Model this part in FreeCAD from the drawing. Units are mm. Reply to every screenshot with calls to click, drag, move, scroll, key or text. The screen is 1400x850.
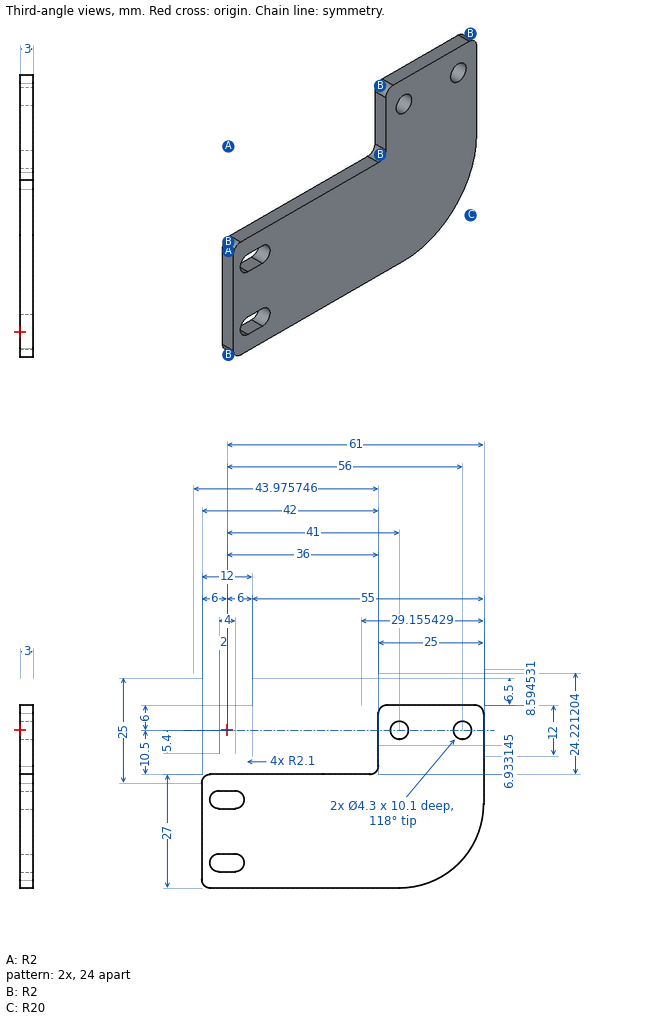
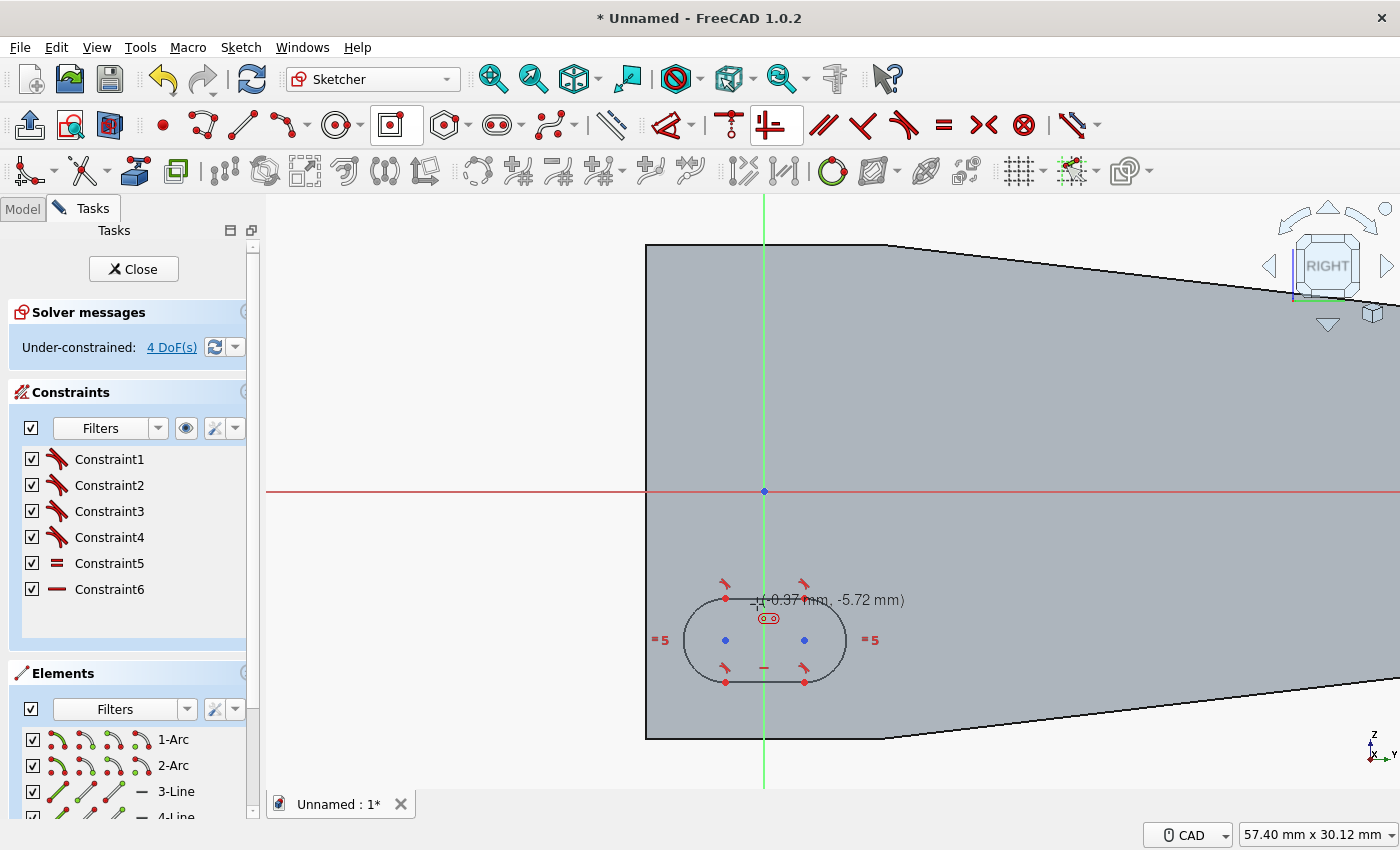
click(725, 344)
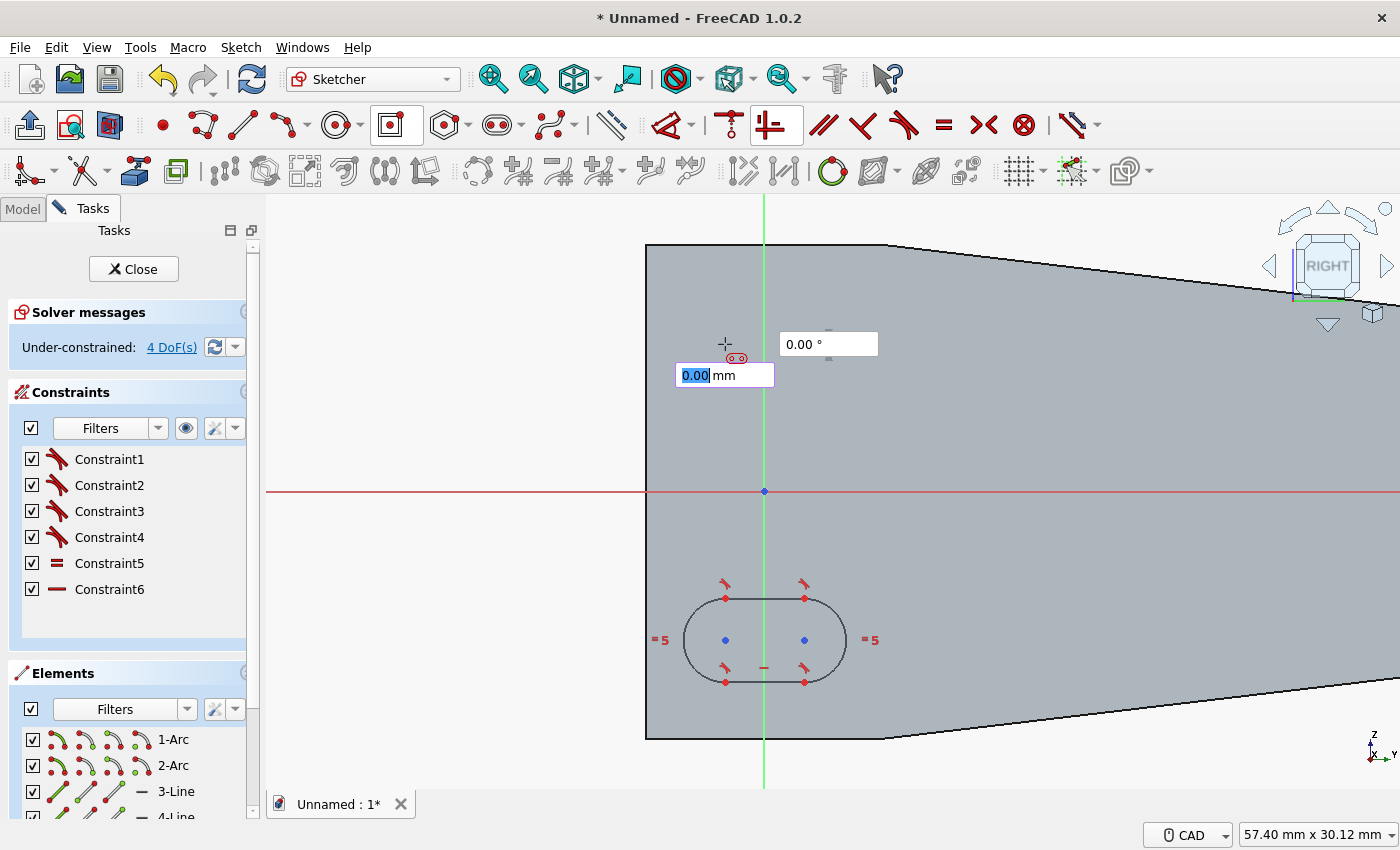
click(804, 344)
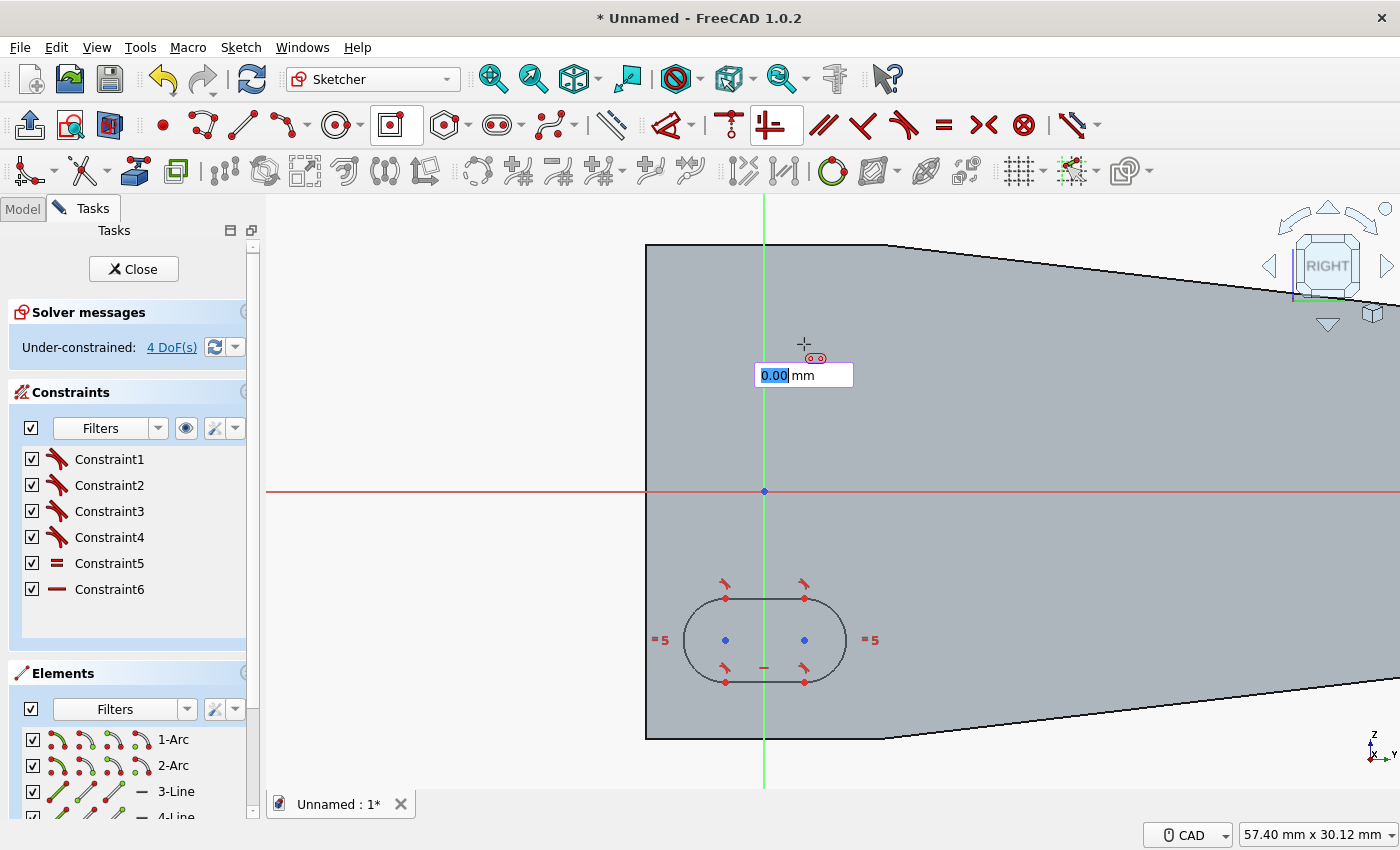
scroll(776, 385, up, 2)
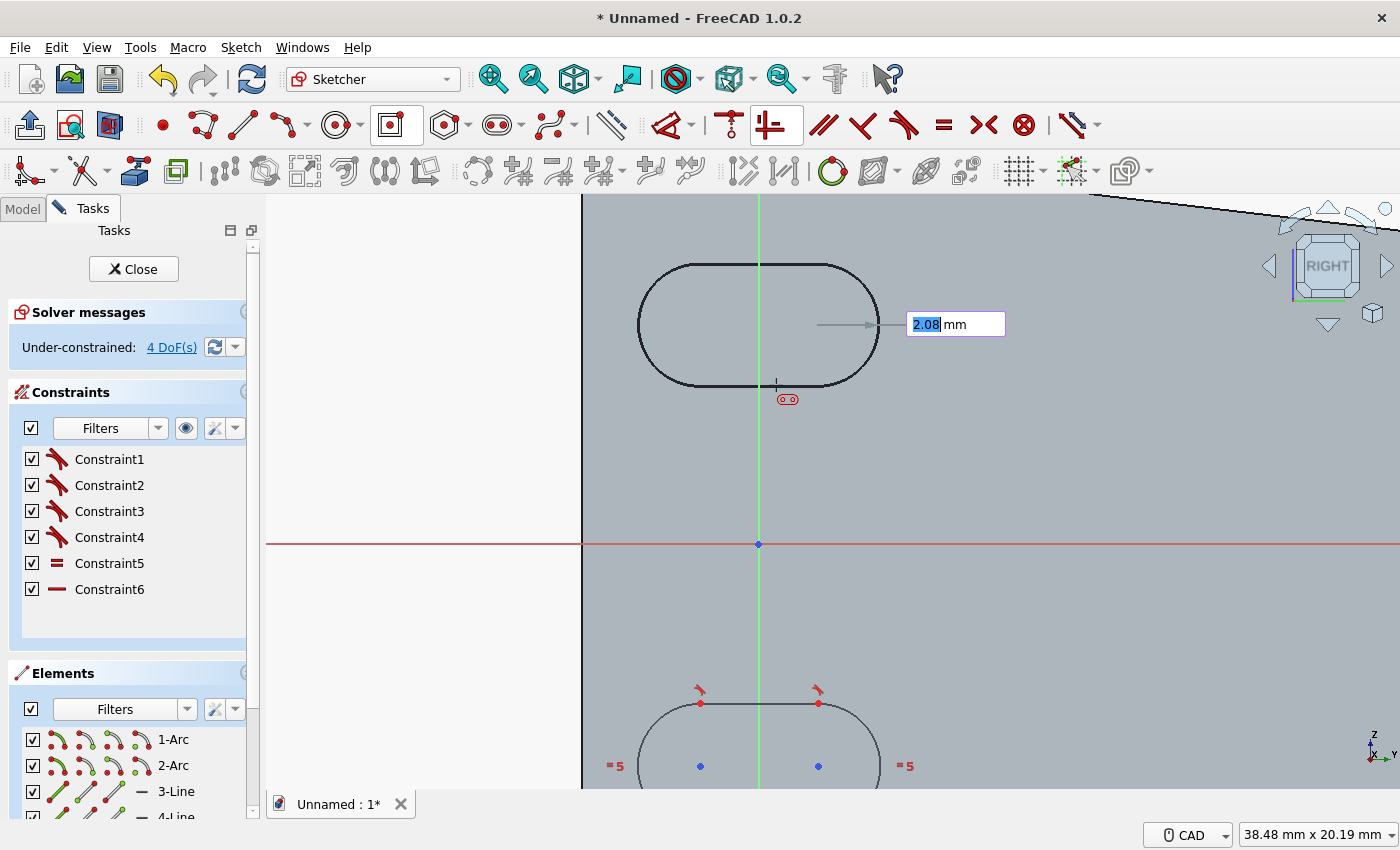
click(776, 385)
key(Escape)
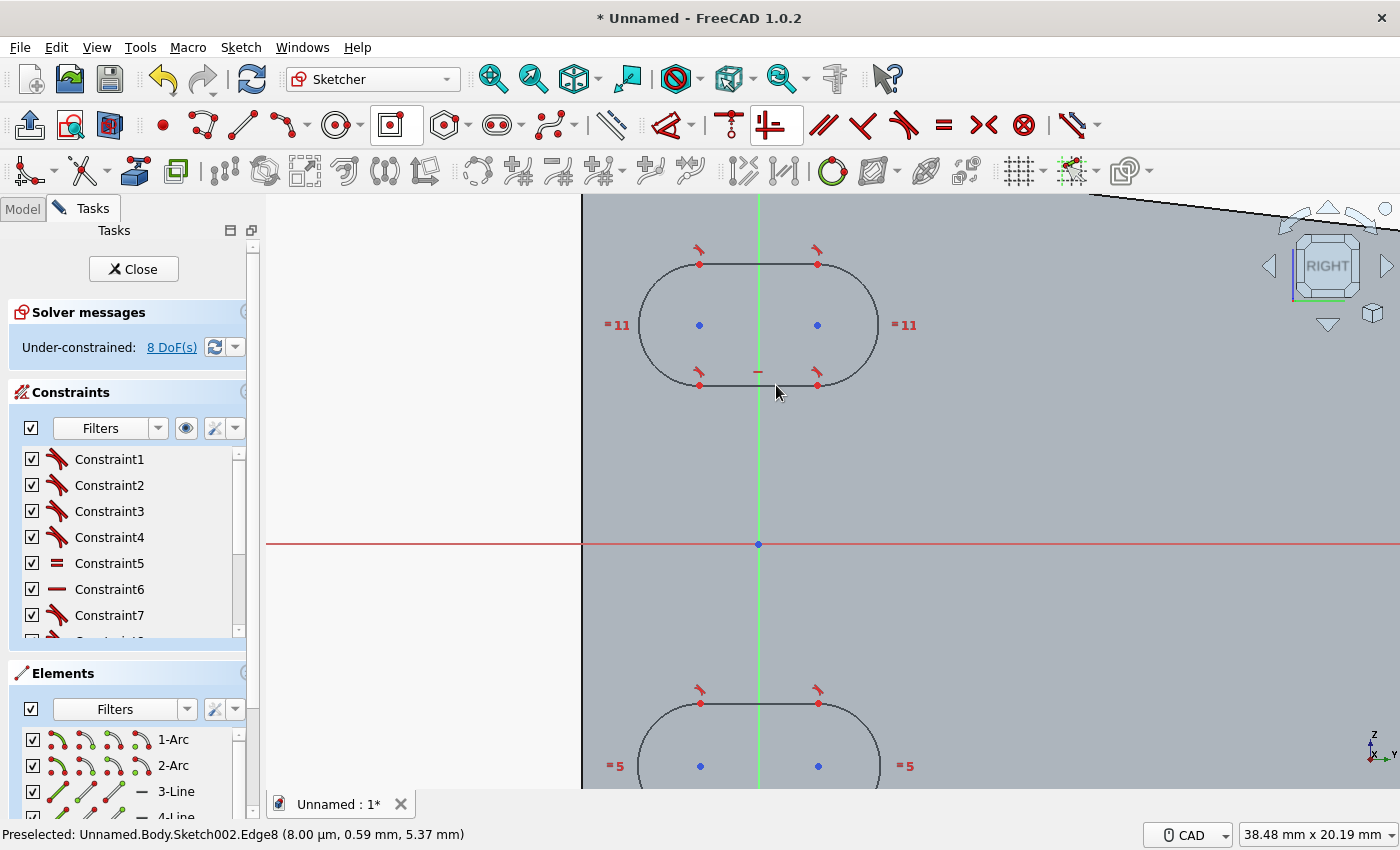
click(650, 730)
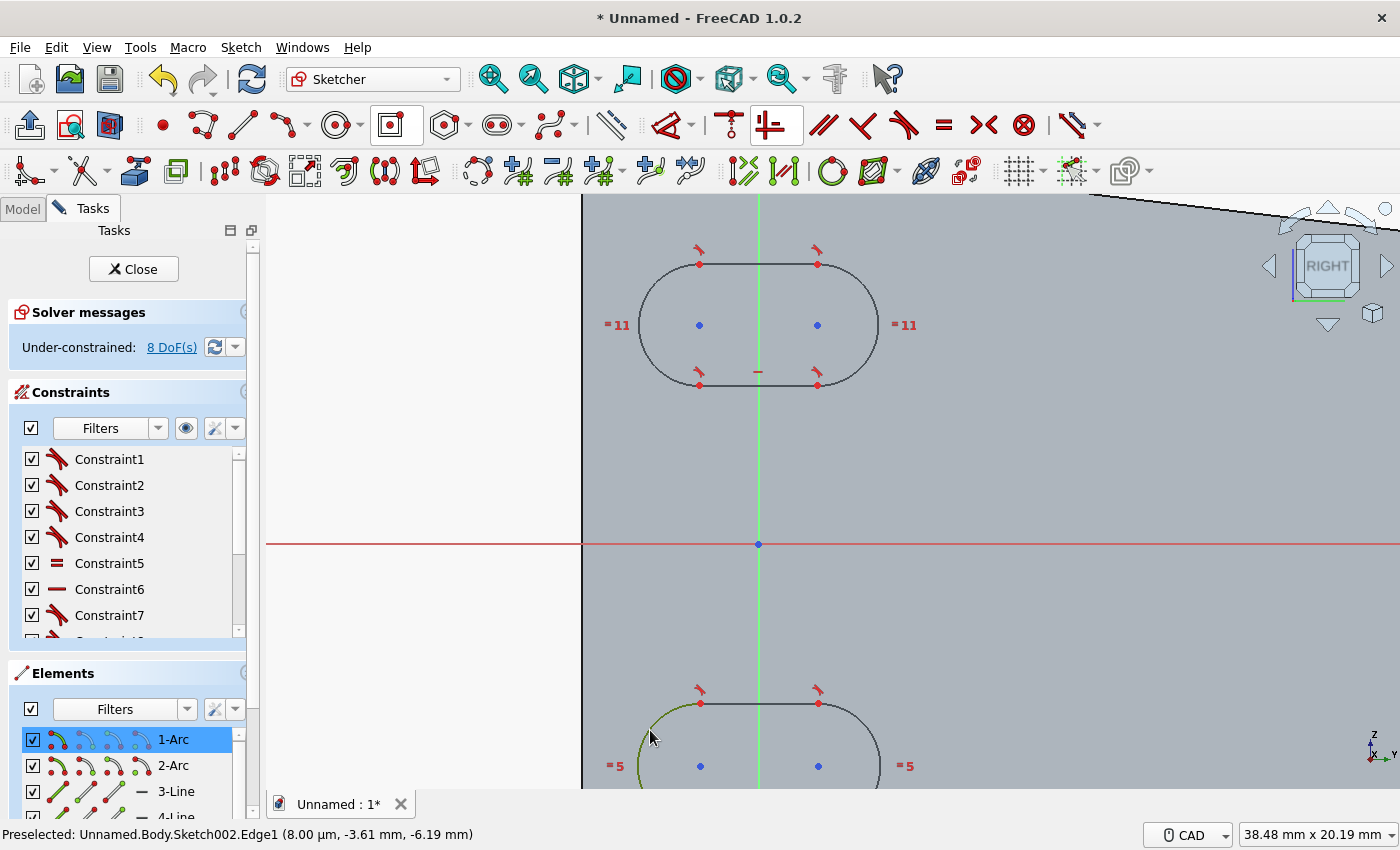
click(650, 289)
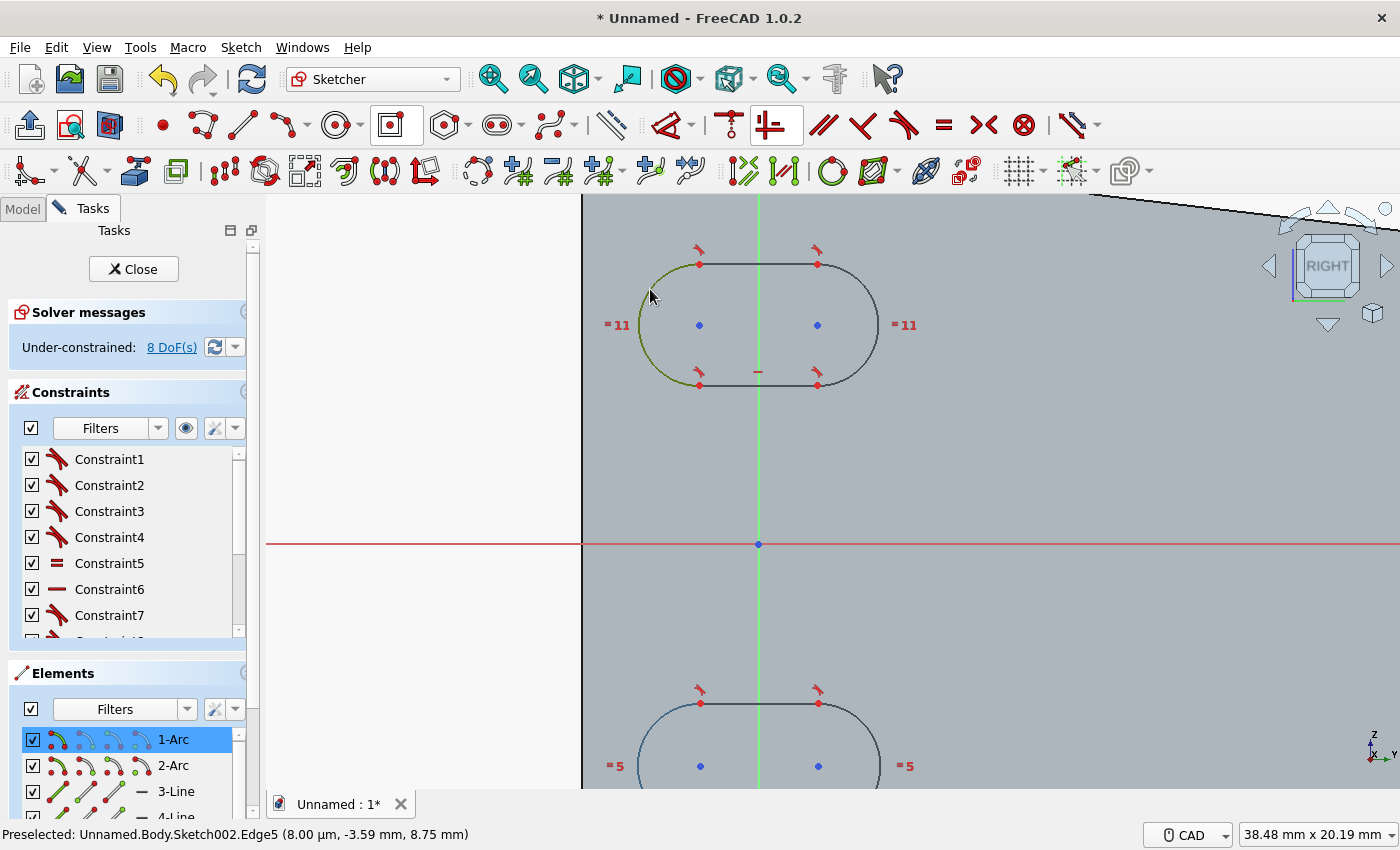
click(944, 126)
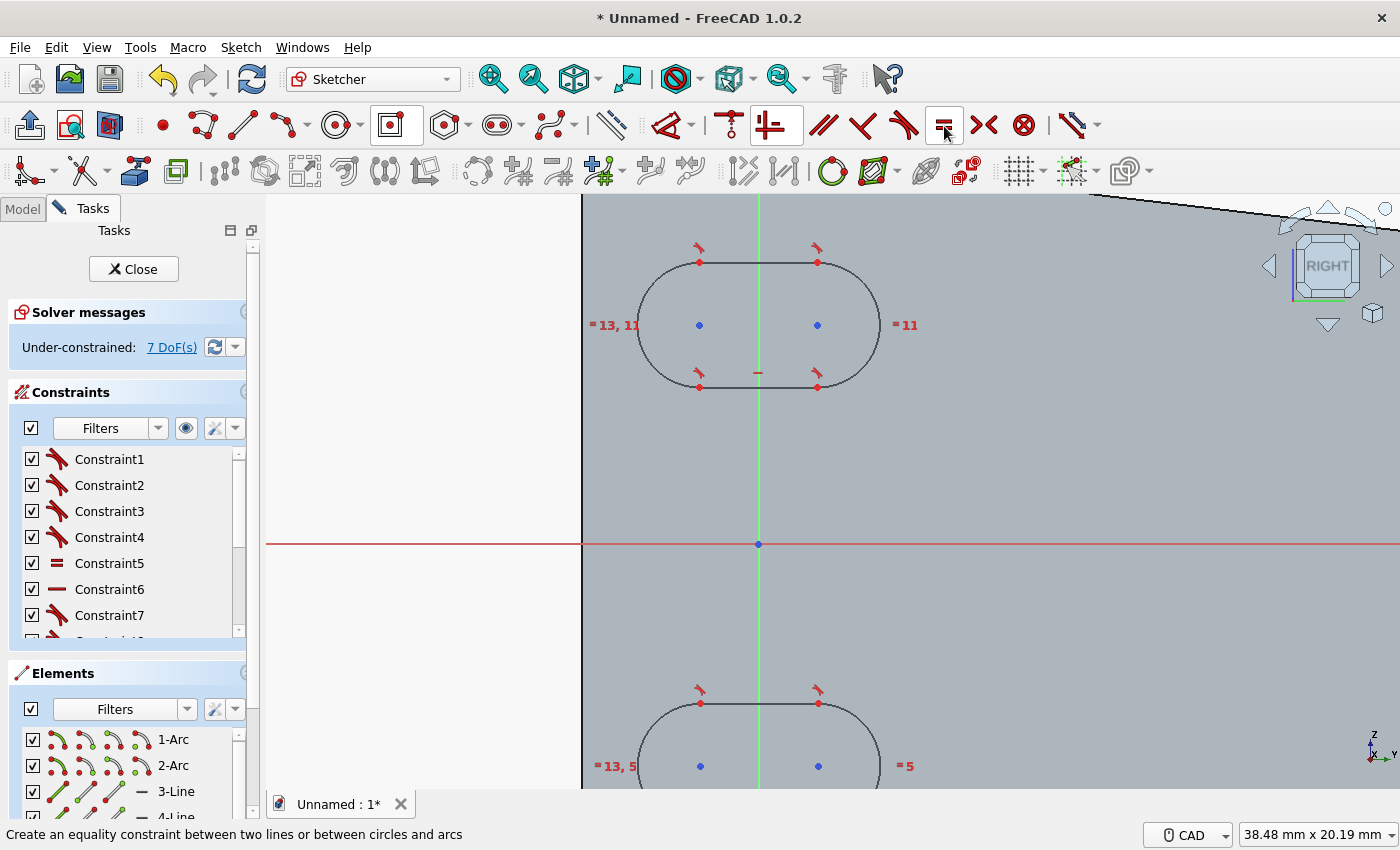
scroll(776, 384, down, 2)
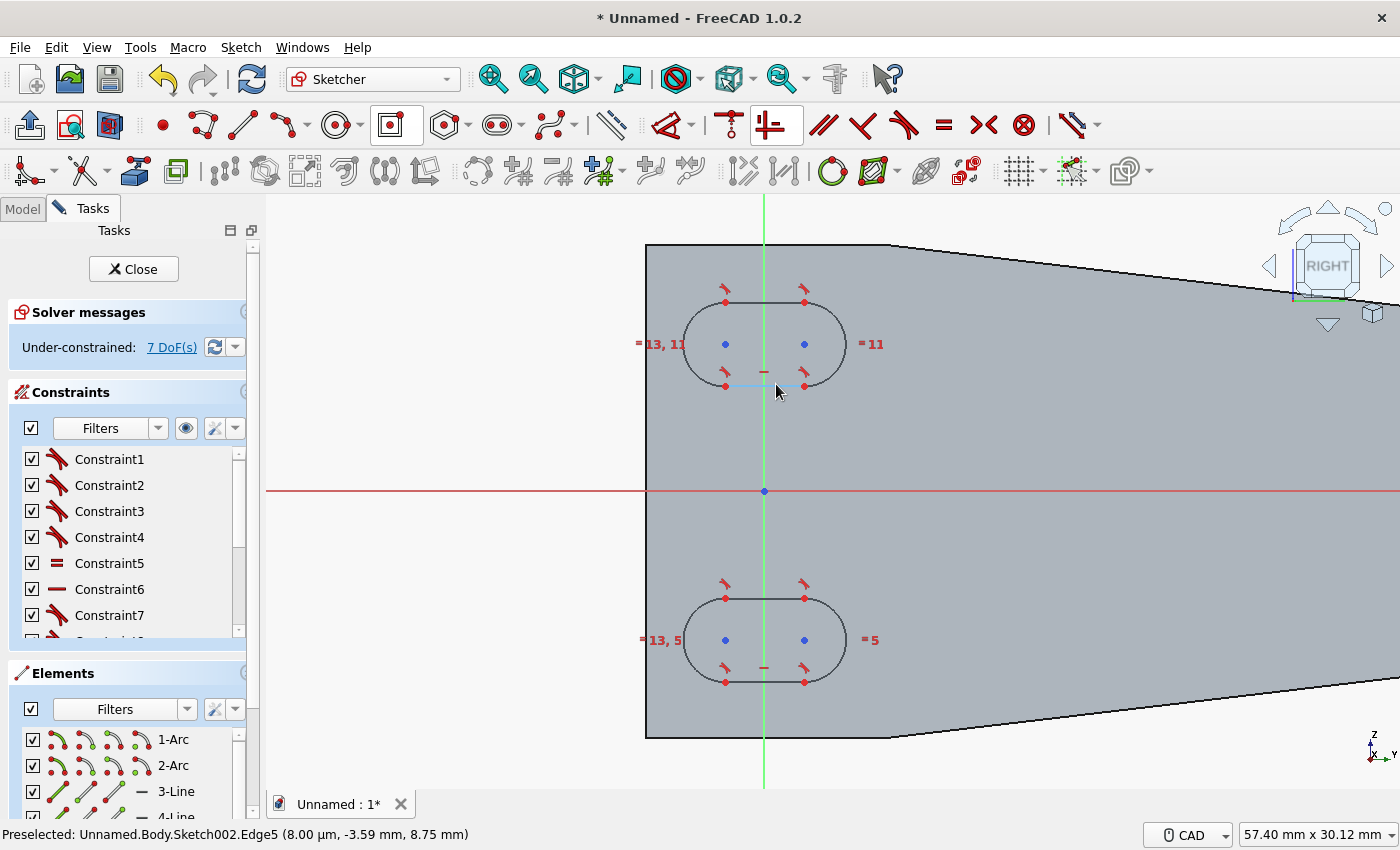
click(725, 640)